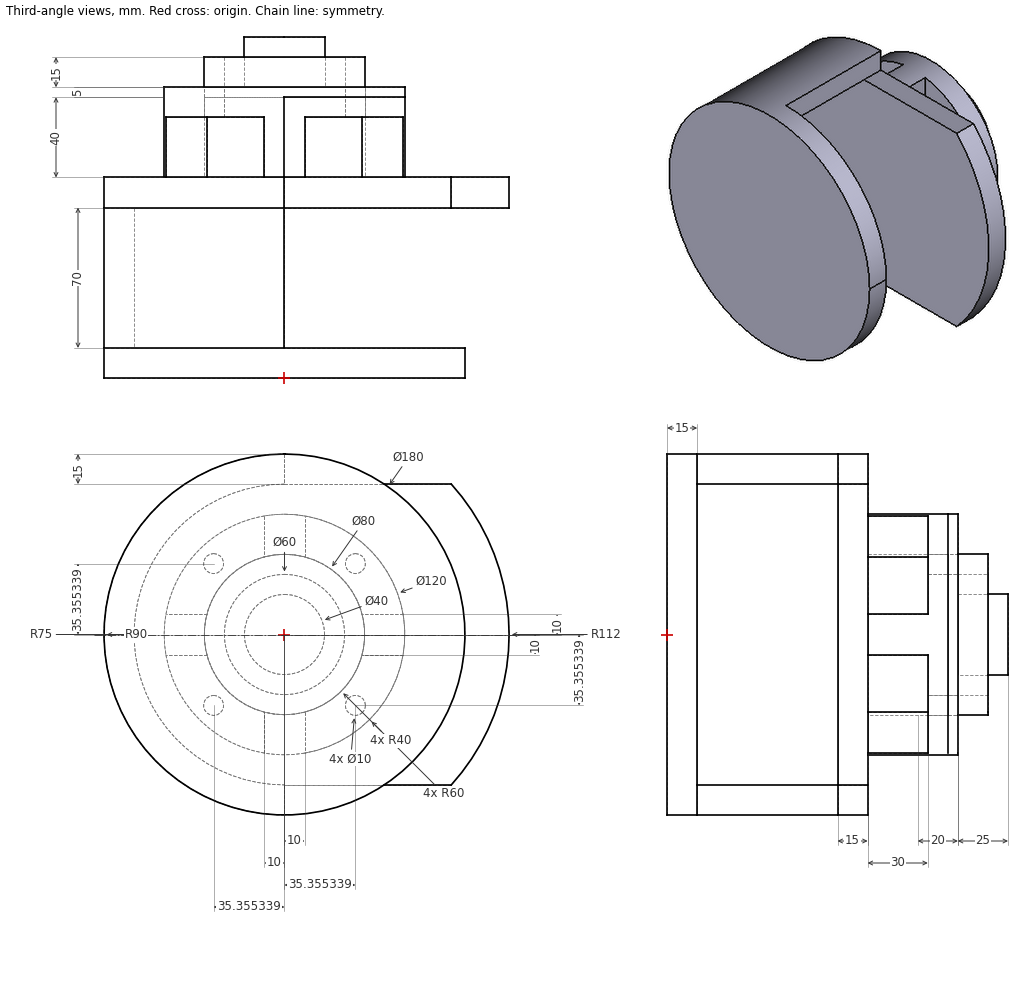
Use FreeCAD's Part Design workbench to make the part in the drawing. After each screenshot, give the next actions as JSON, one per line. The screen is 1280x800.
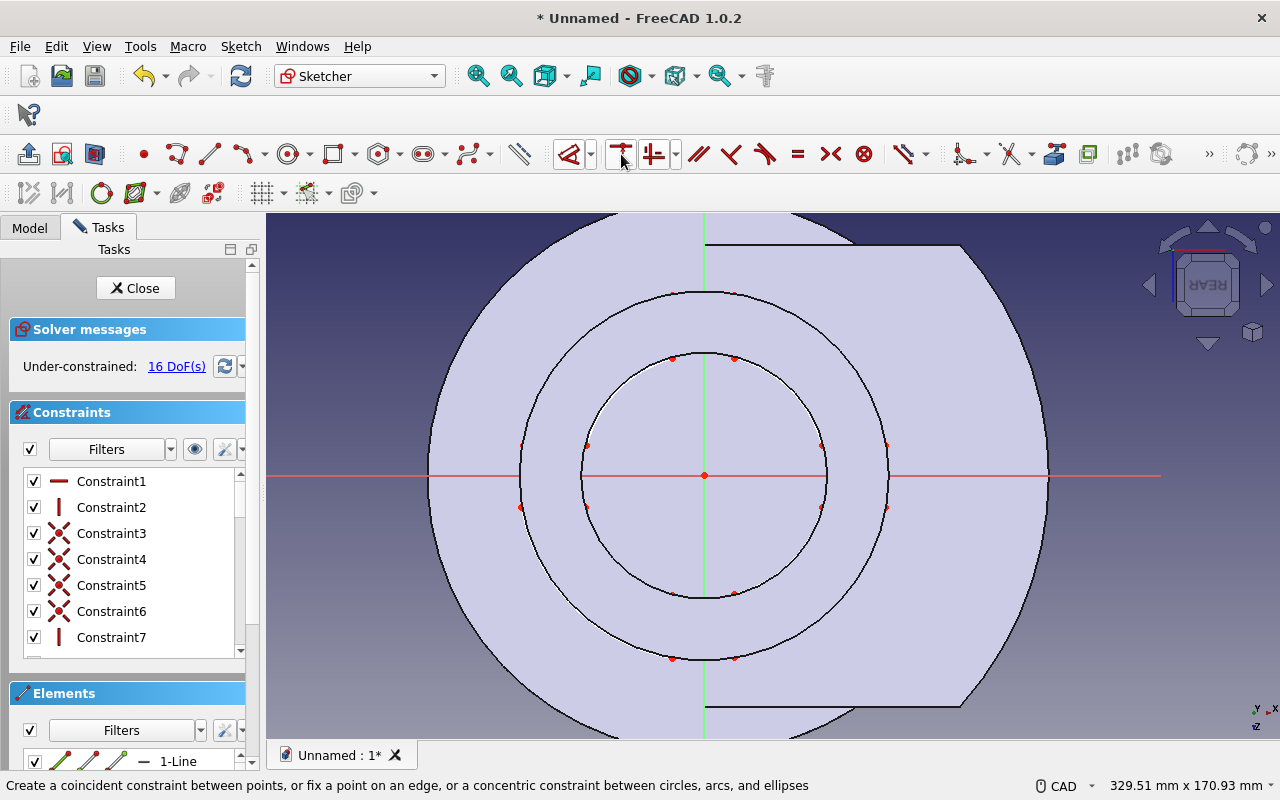
{"action": "left_click", "coordinate": [862, 382]}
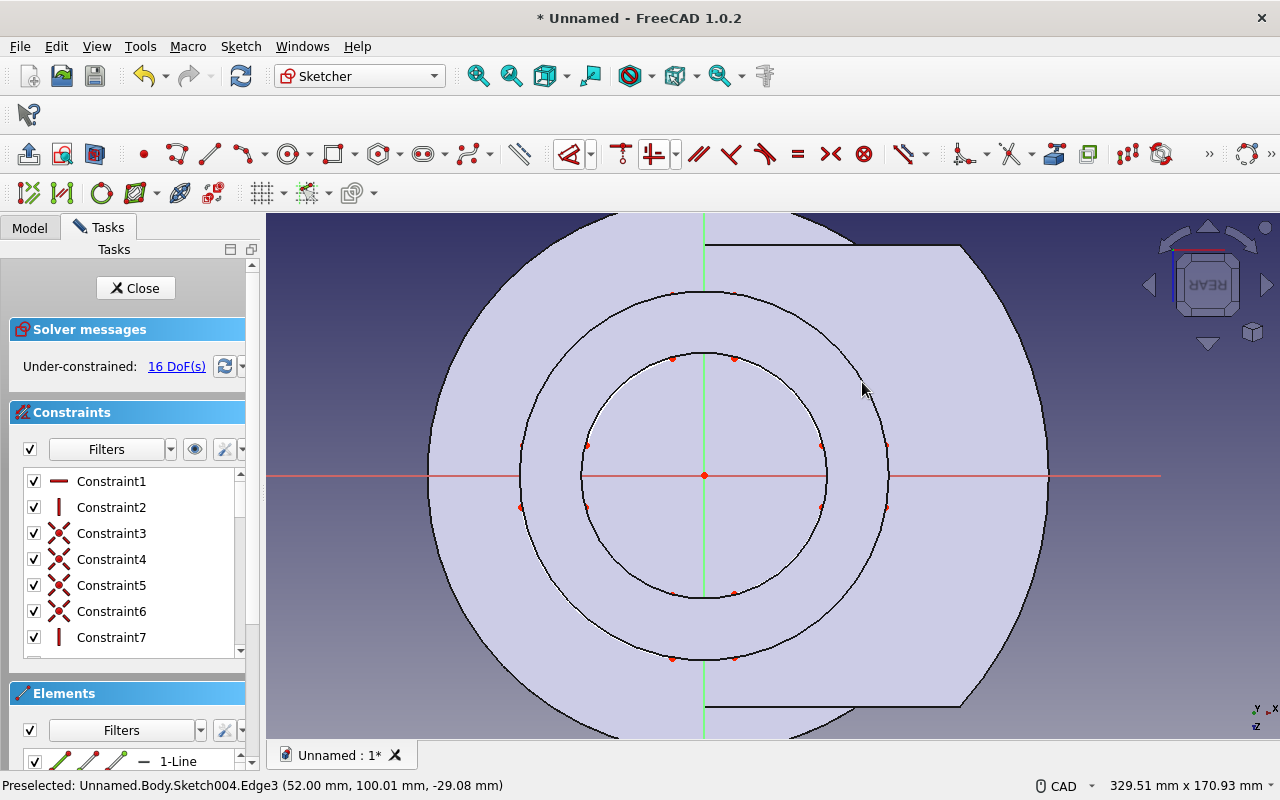
{"action": "left_click", "coordinate": [610, 319]}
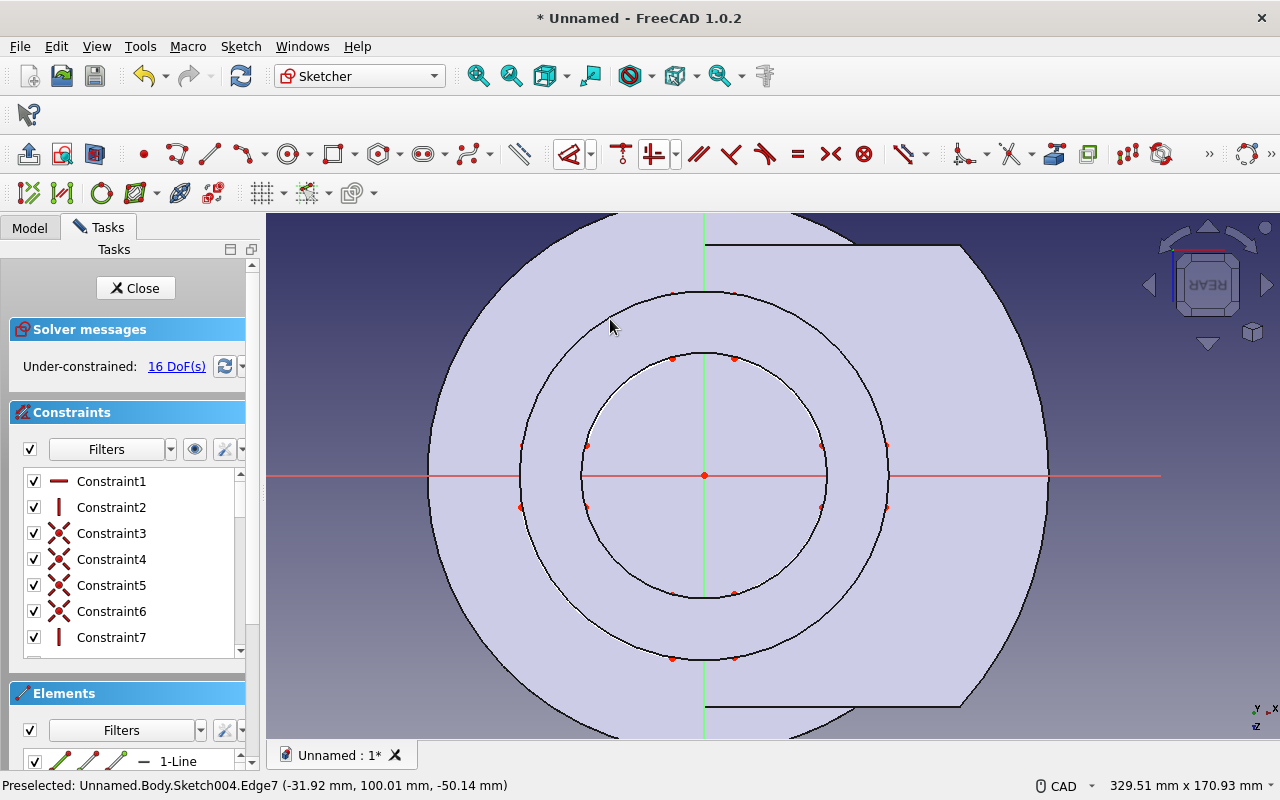
{"action": "left_click", "coordinate": [798, 634]}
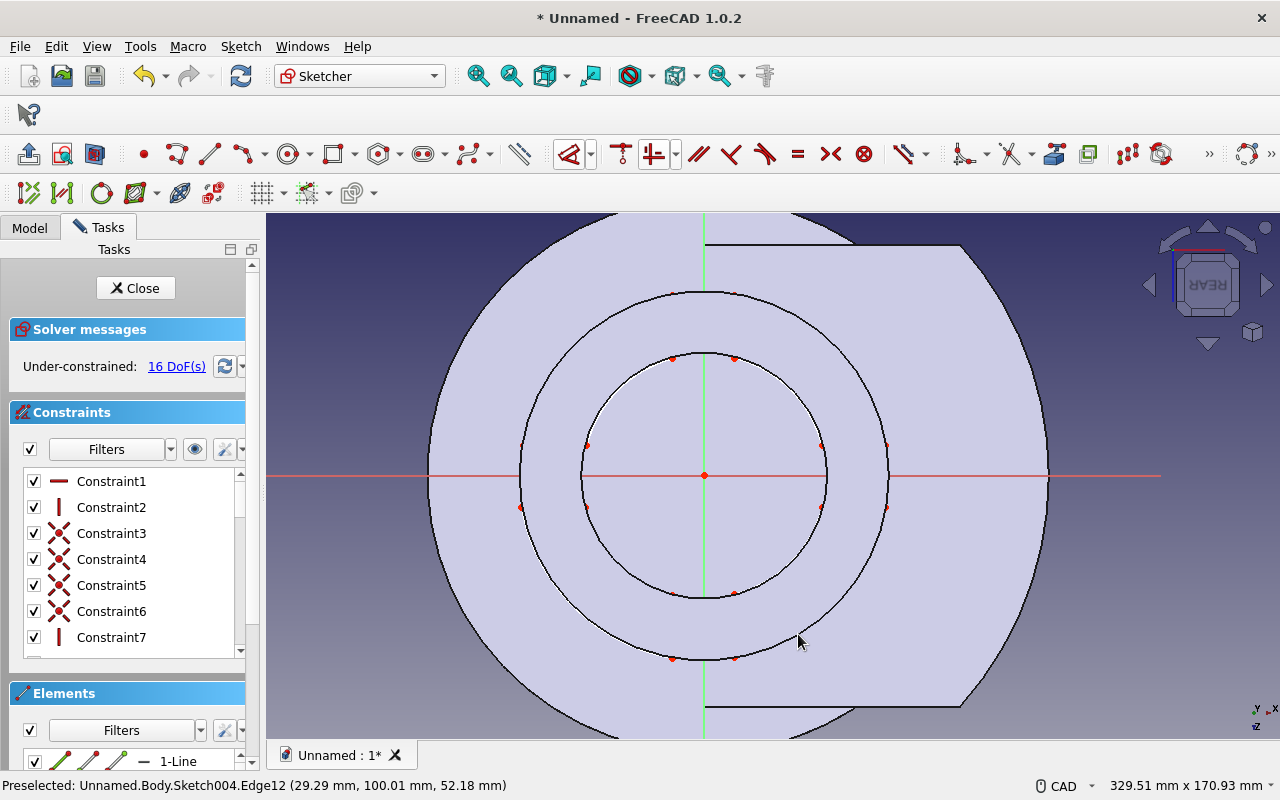
{"action": "left_click", "coordinate": [546, 571]}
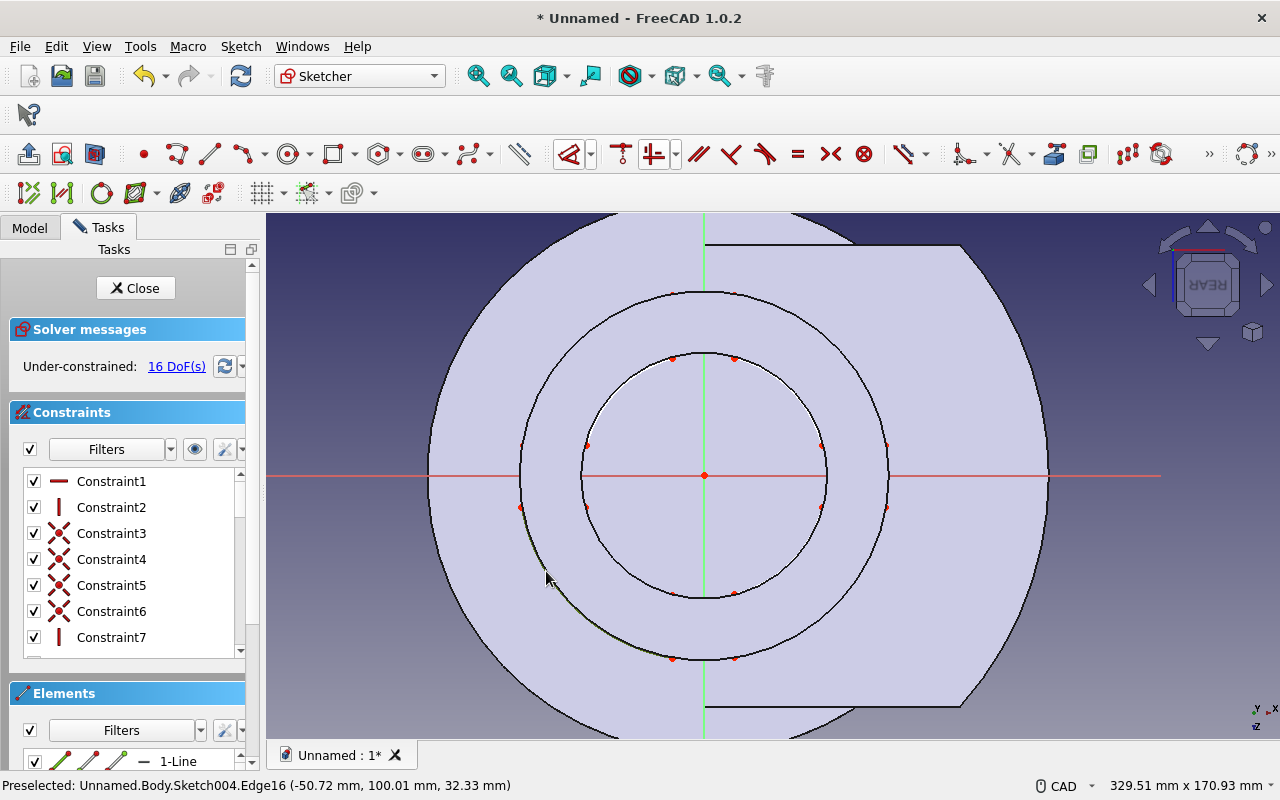
{"action": "left_click", "coordinate": [798, 154]}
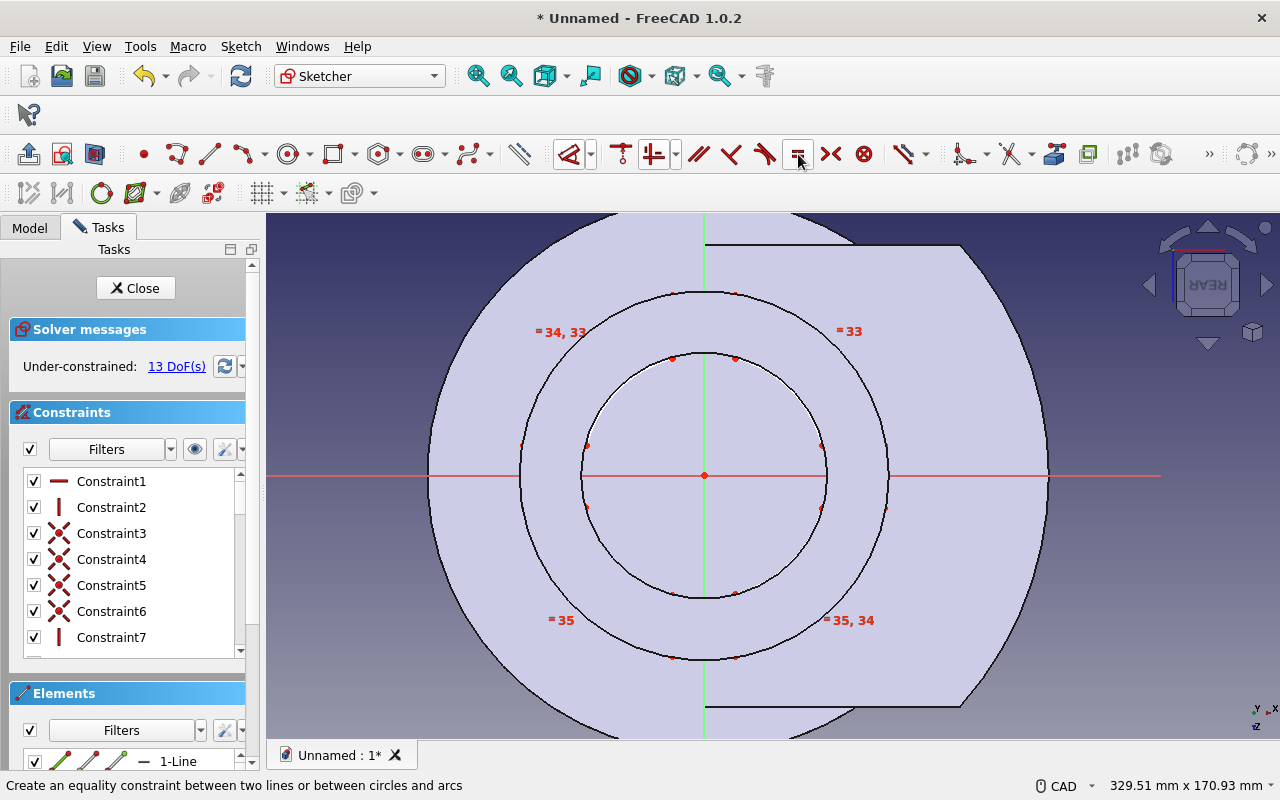
{"action": "left_click", "coordinate": [807, 410]}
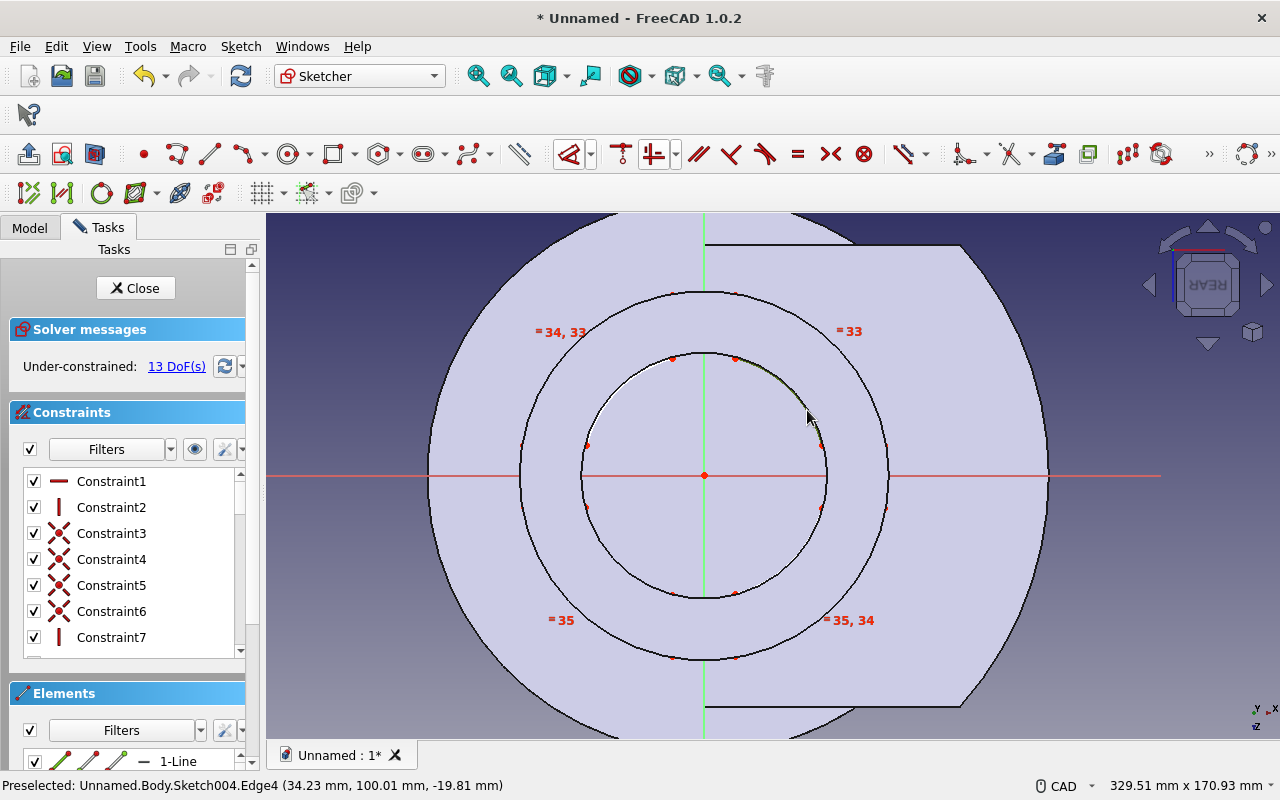
{"action": "left_click", "coordinate": [638, 374]}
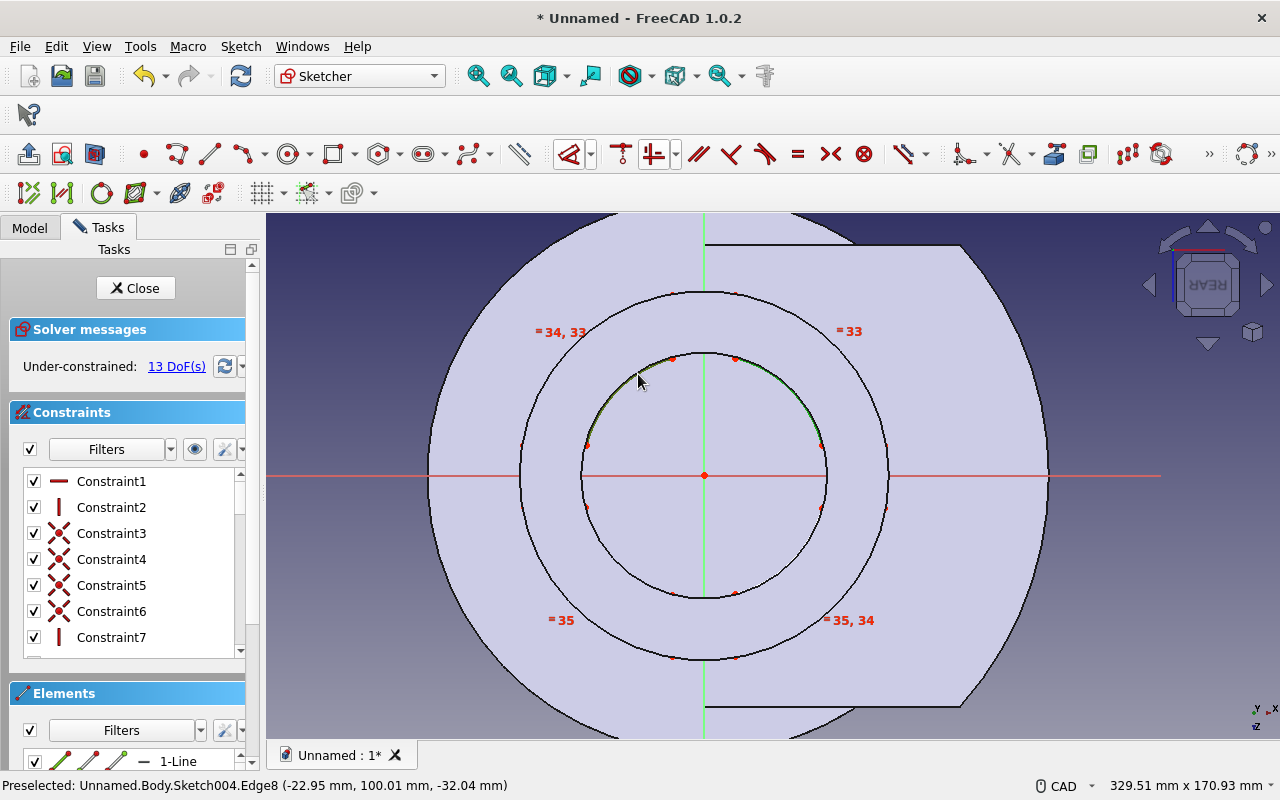
{"action": "left_click", "coordinate": [770, 579]}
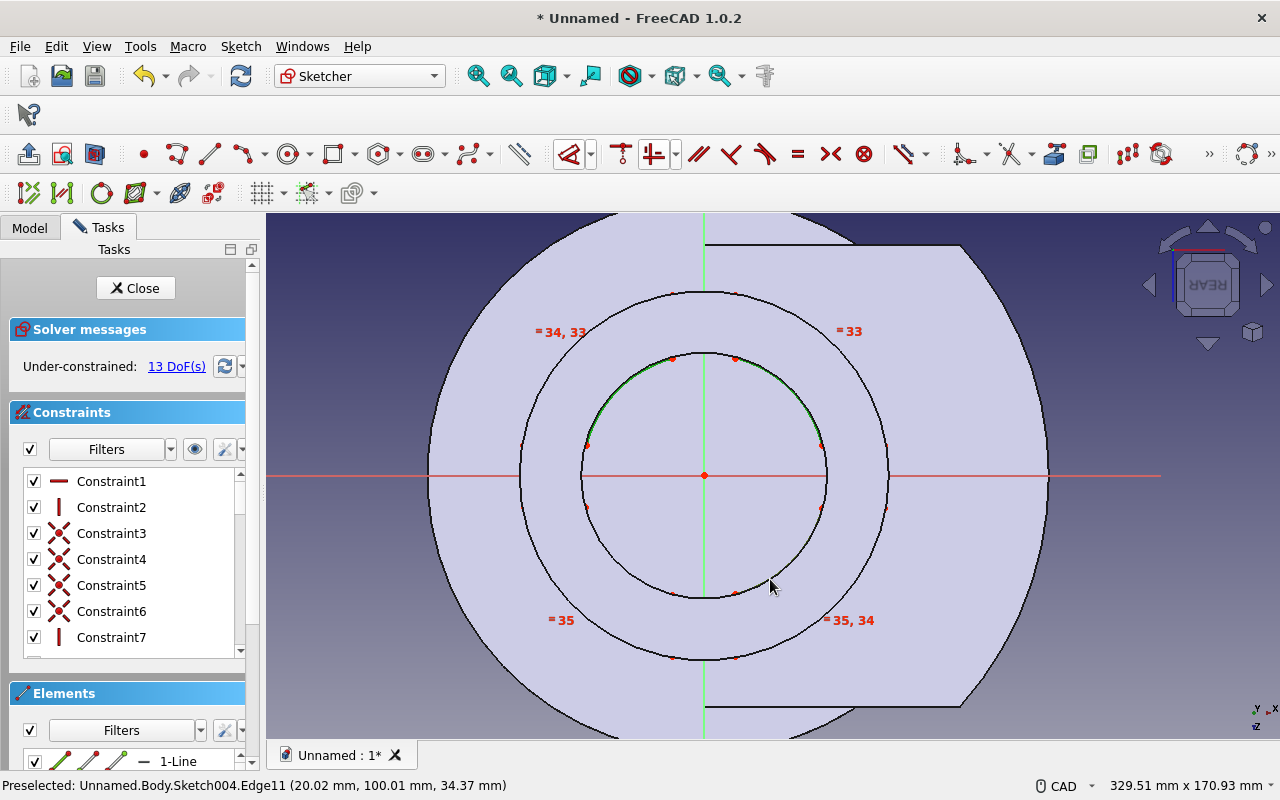
{"action": "left_click", "coordinate": [601, 543]}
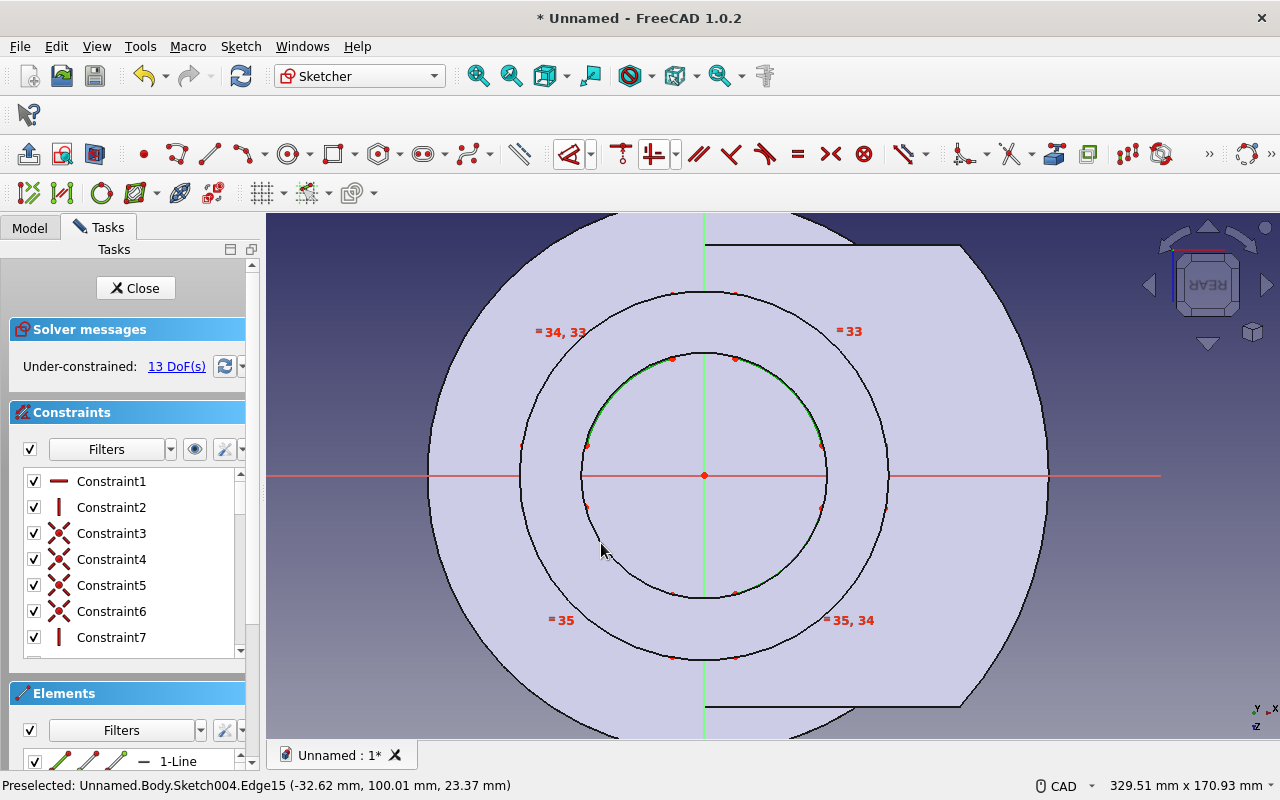
{"action": "left_click", "coordinate": [798, 154]}